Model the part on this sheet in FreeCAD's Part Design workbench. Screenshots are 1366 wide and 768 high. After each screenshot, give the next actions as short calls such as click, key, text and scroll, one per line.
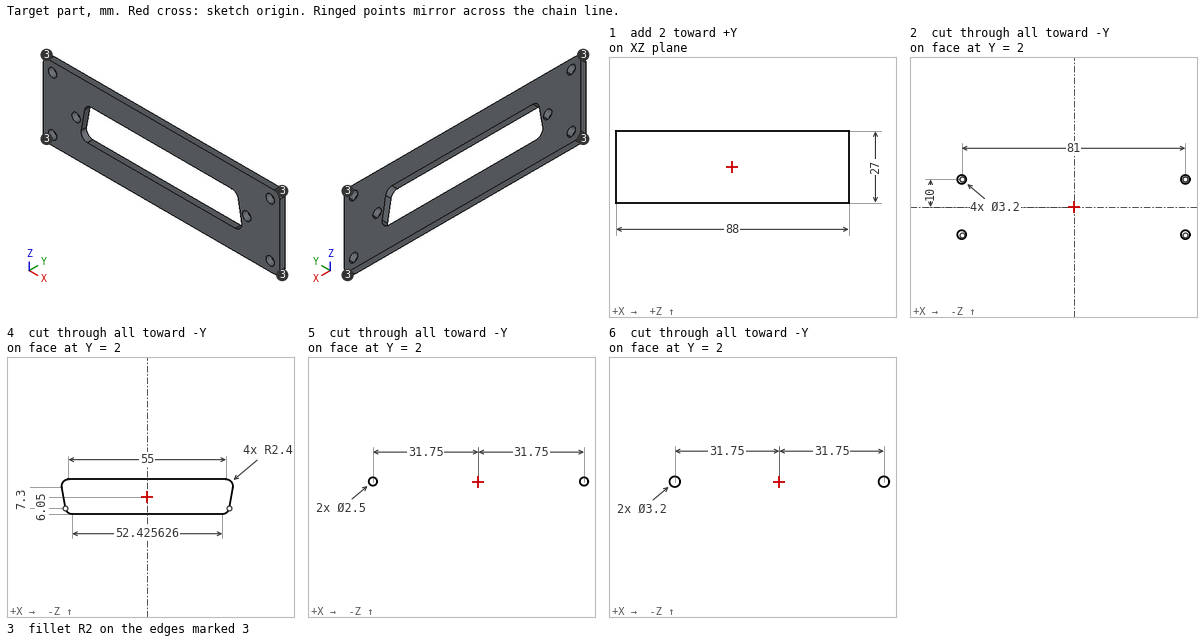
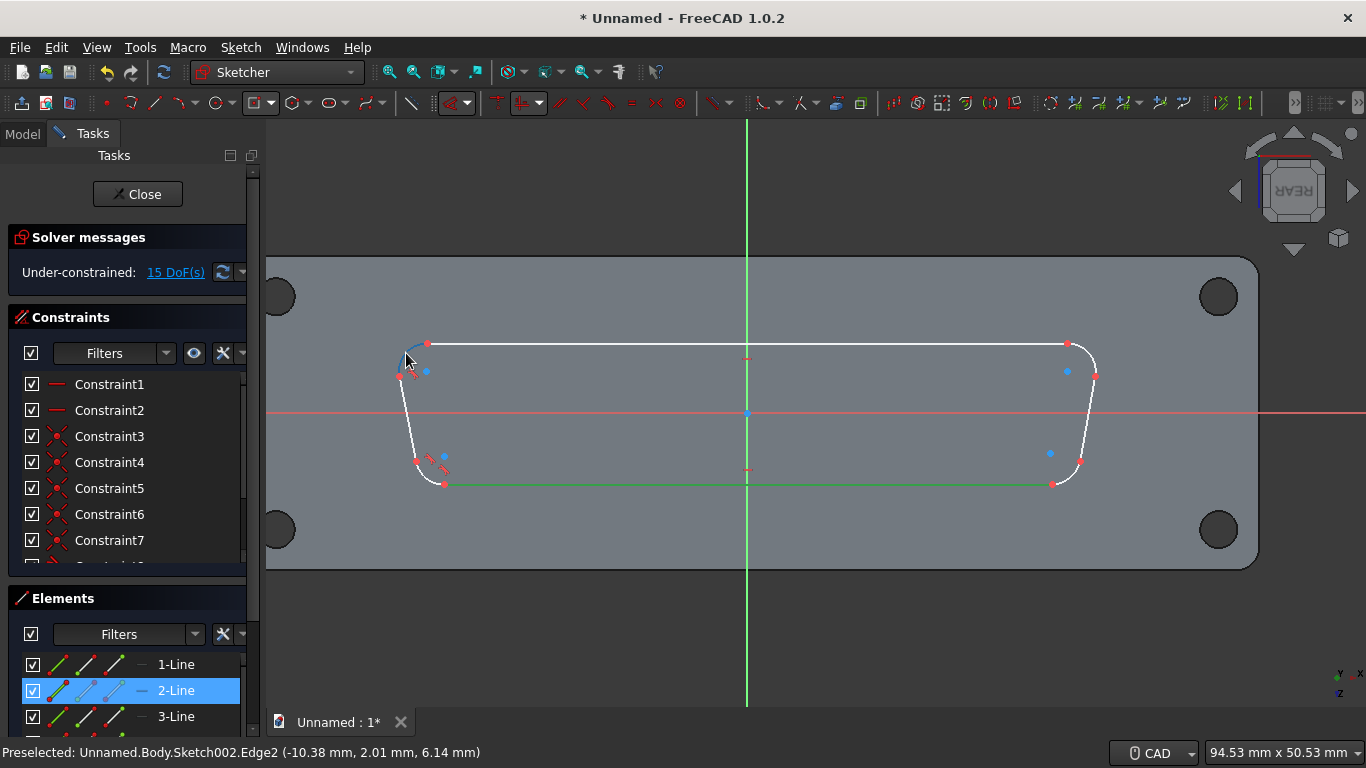
click(1063, 482)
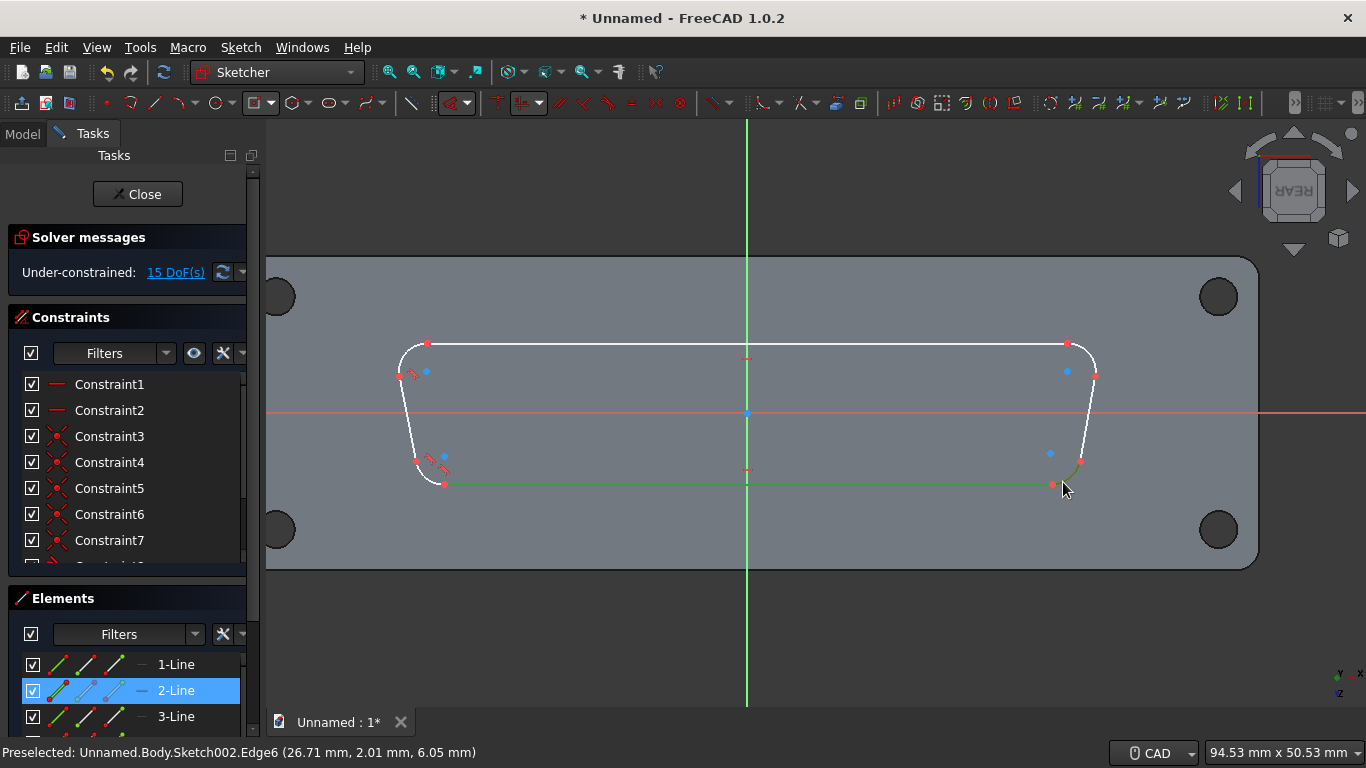
click(608, 104)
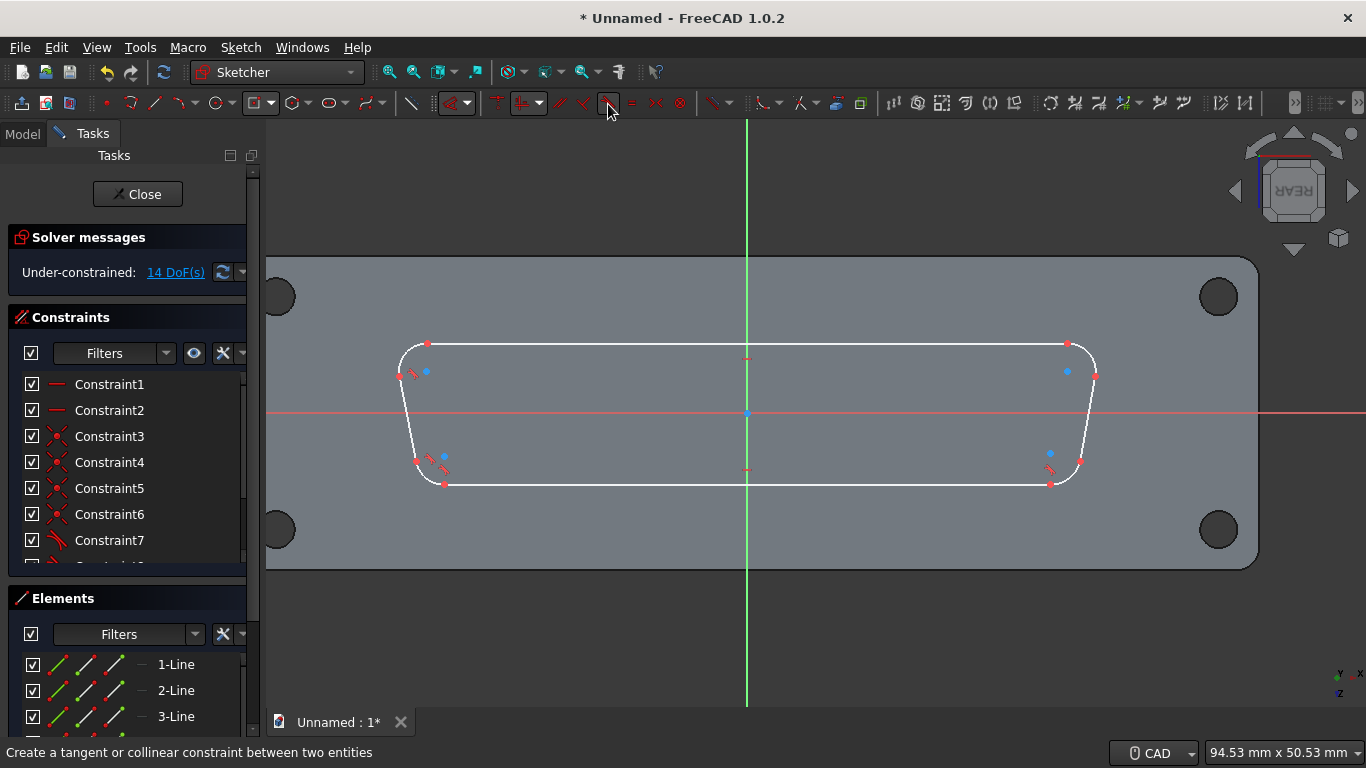
click(1085, 436)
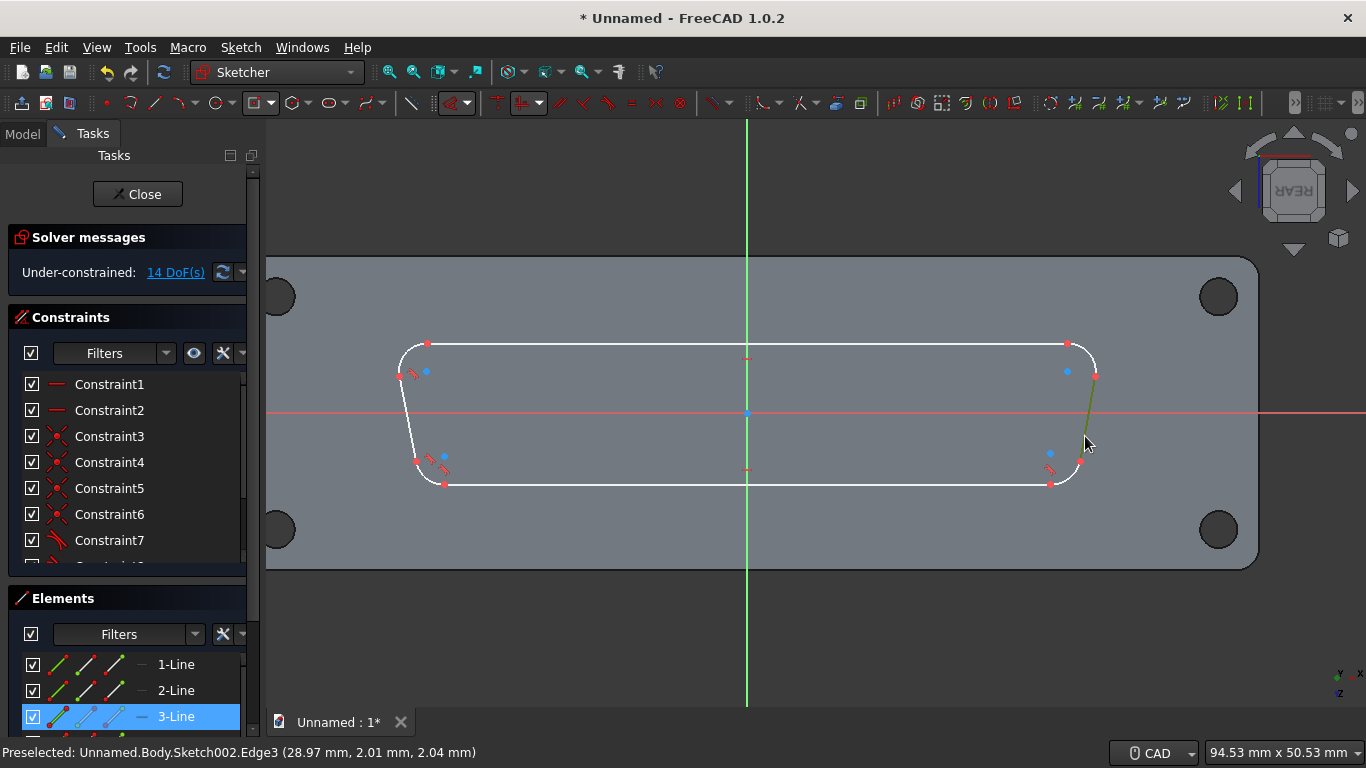
click(1062, 482)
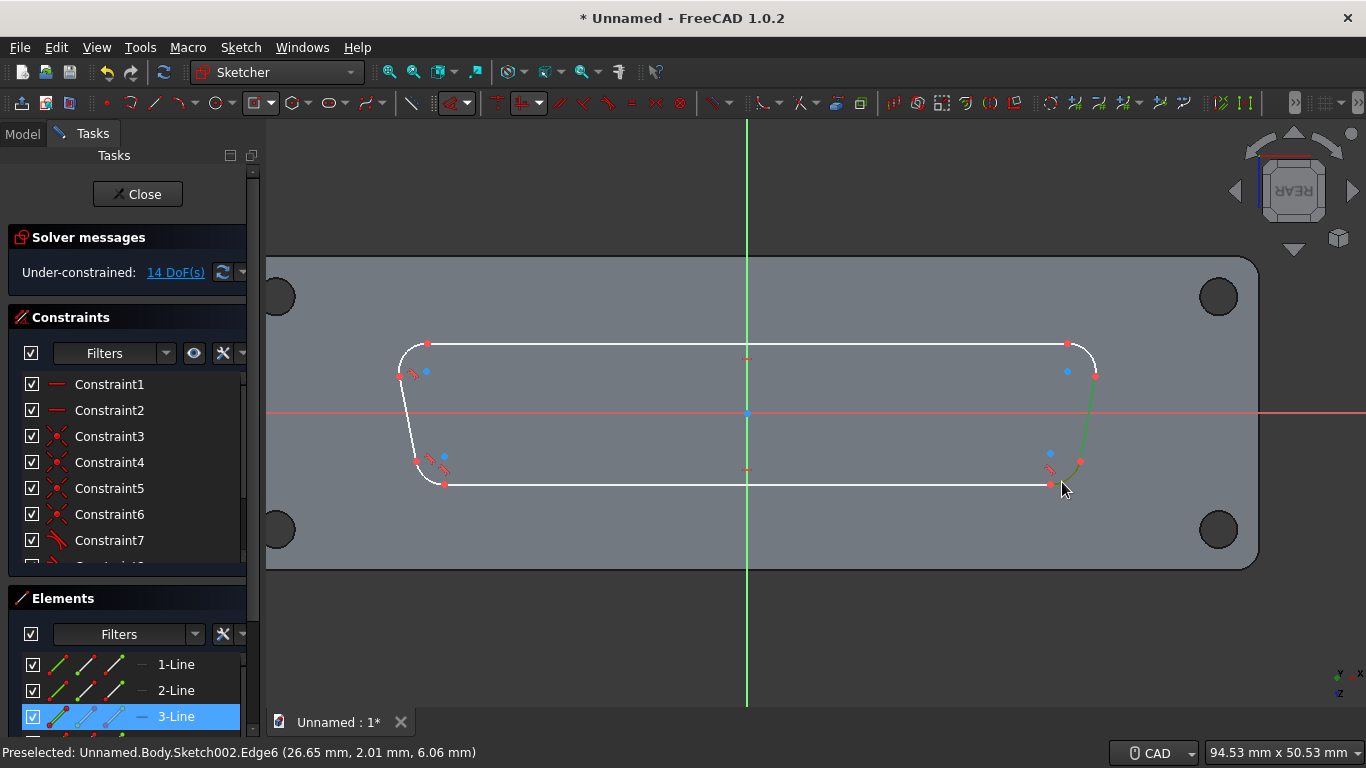
click(608, 104)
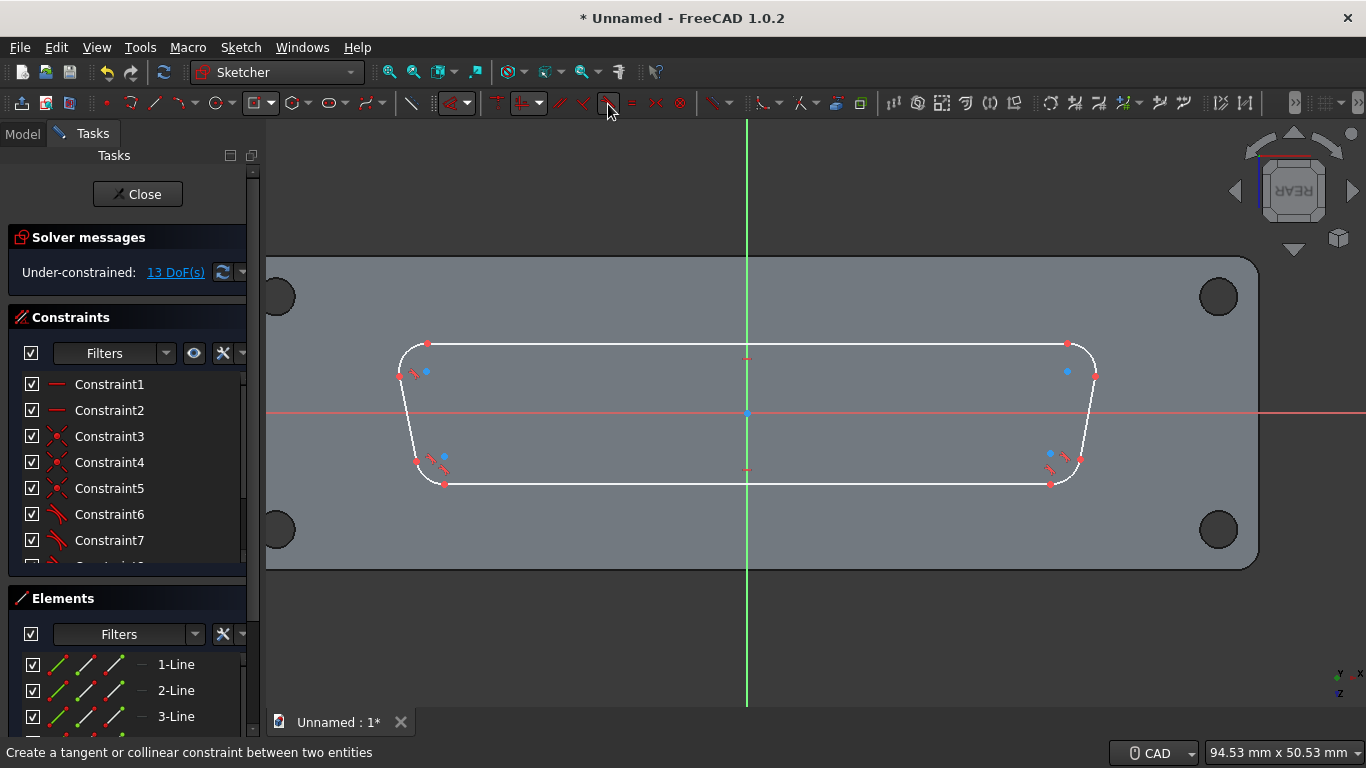
click(1085, 435)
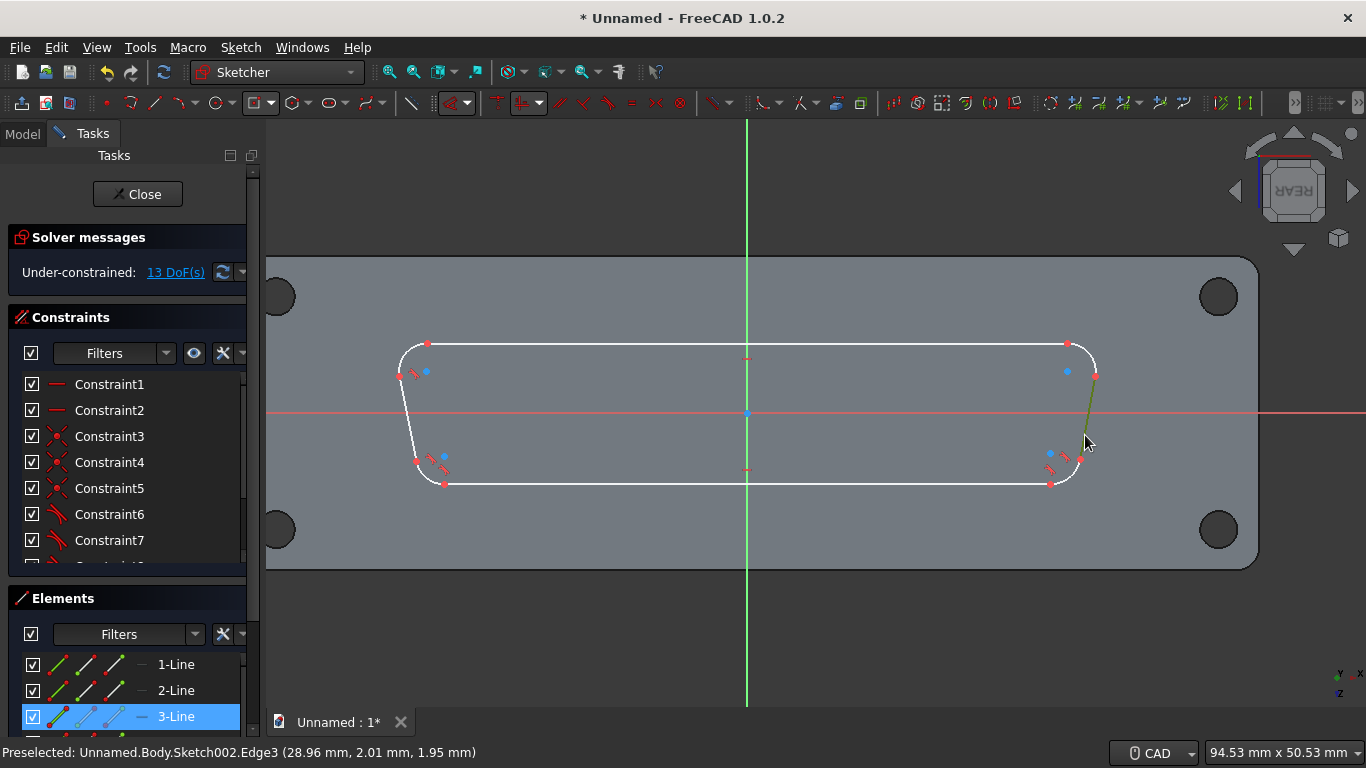
click(1094, 362)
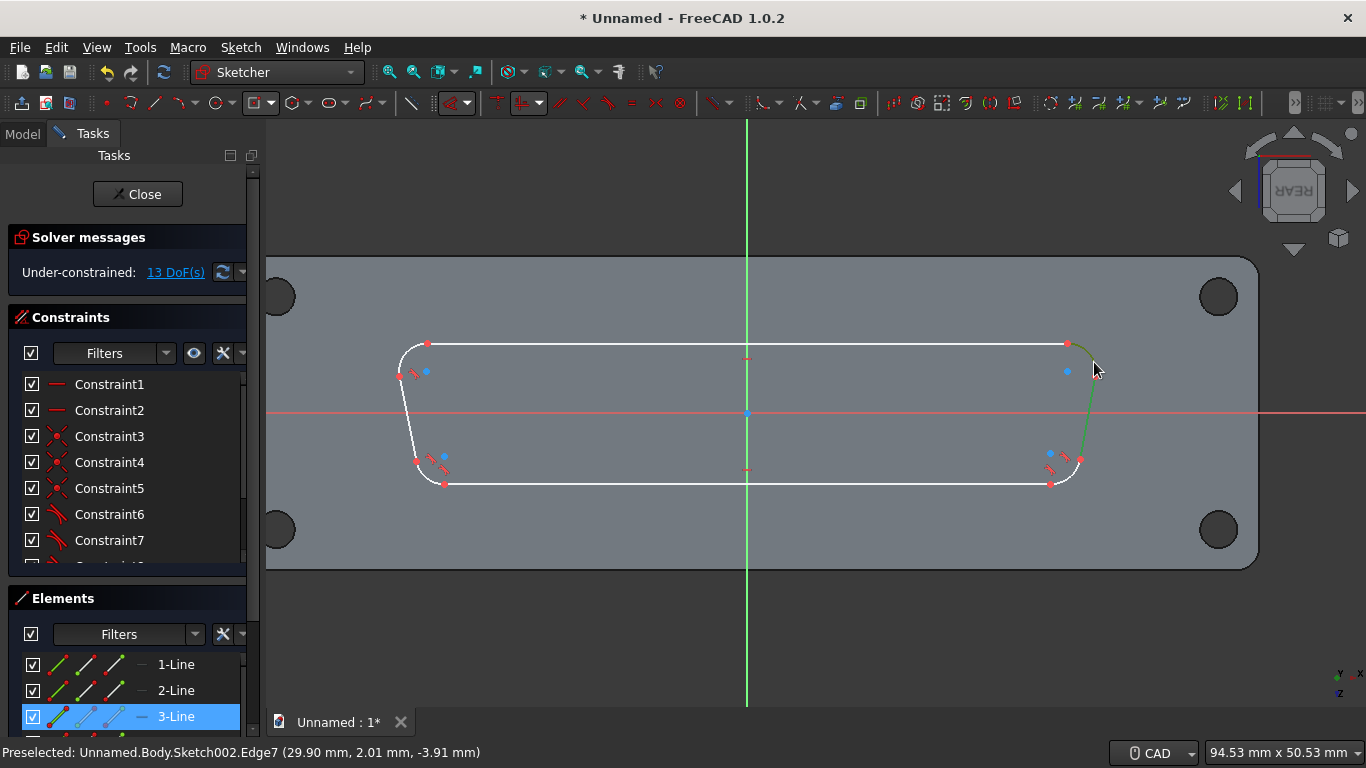
key(t)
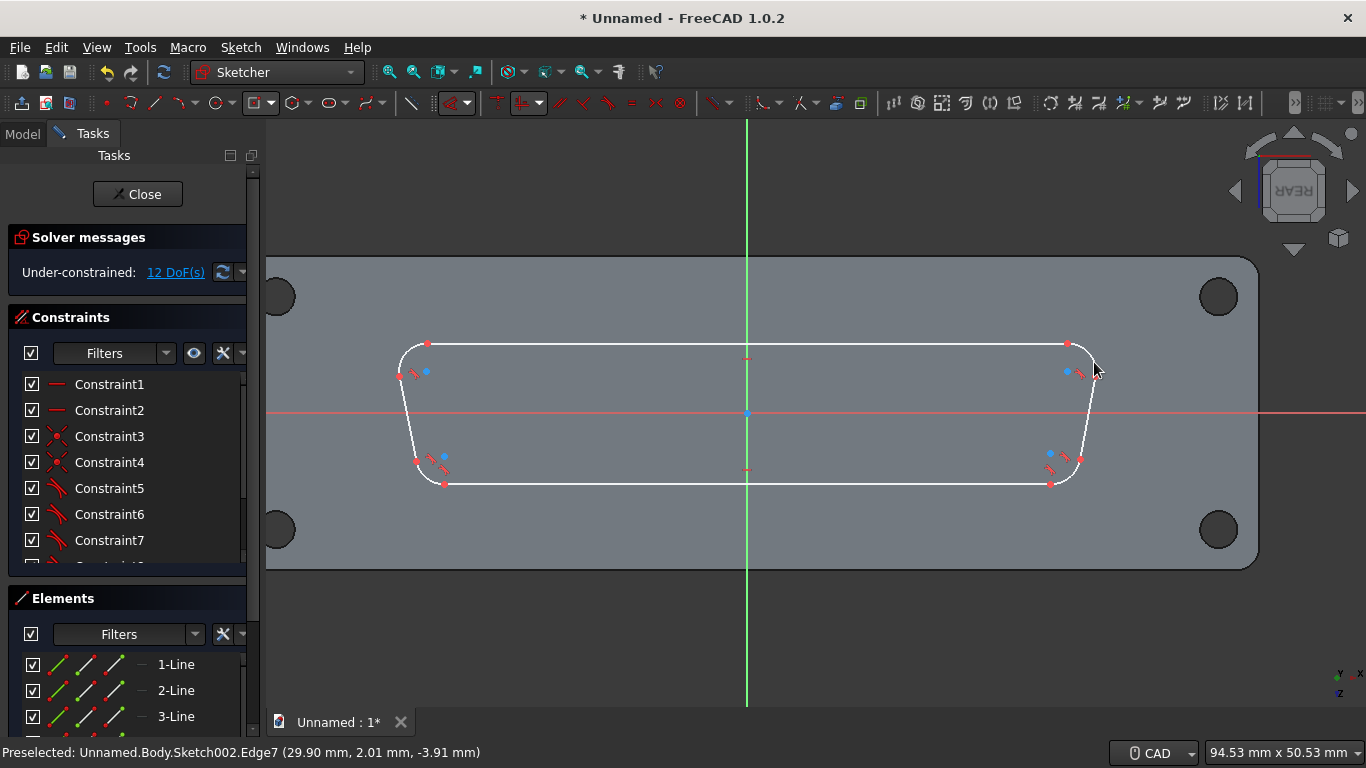
click(875, 344)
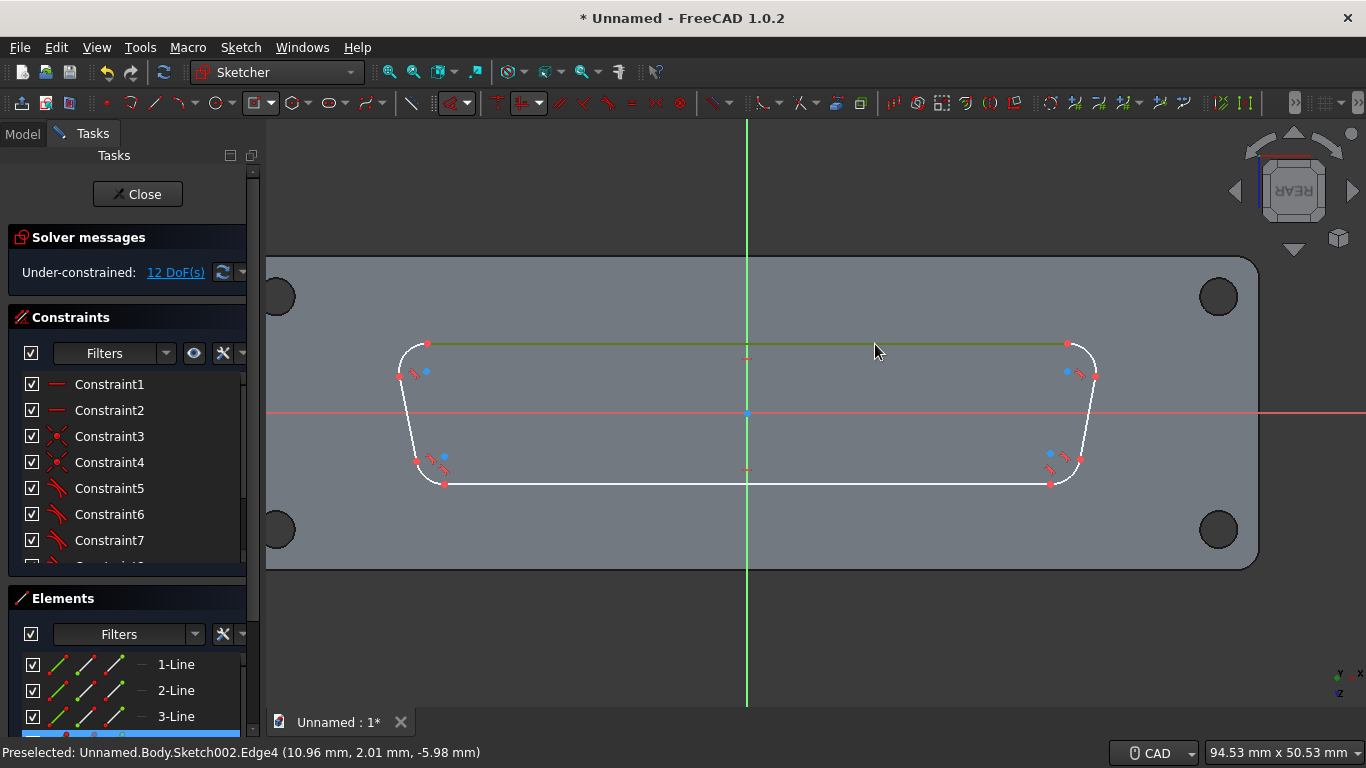
click(1094, 362)